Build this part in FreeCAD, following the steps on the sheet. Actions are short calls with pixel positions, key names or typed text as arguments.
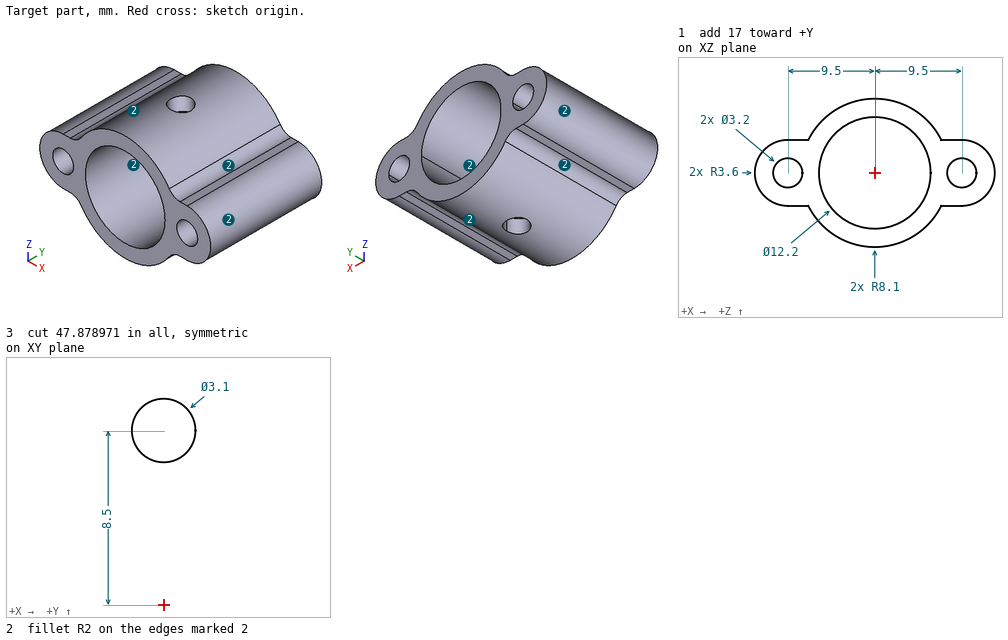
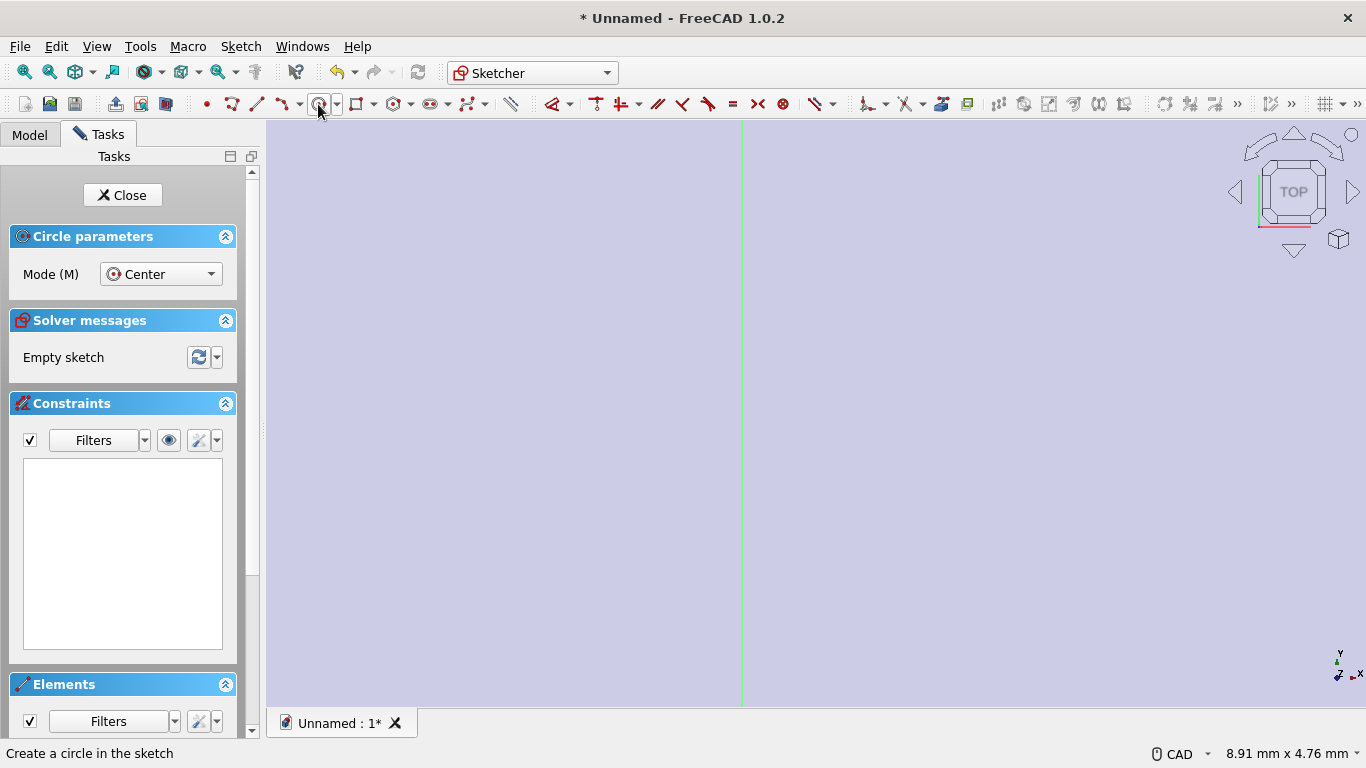
click(742, 407)
click(878, 272)
key(Escape)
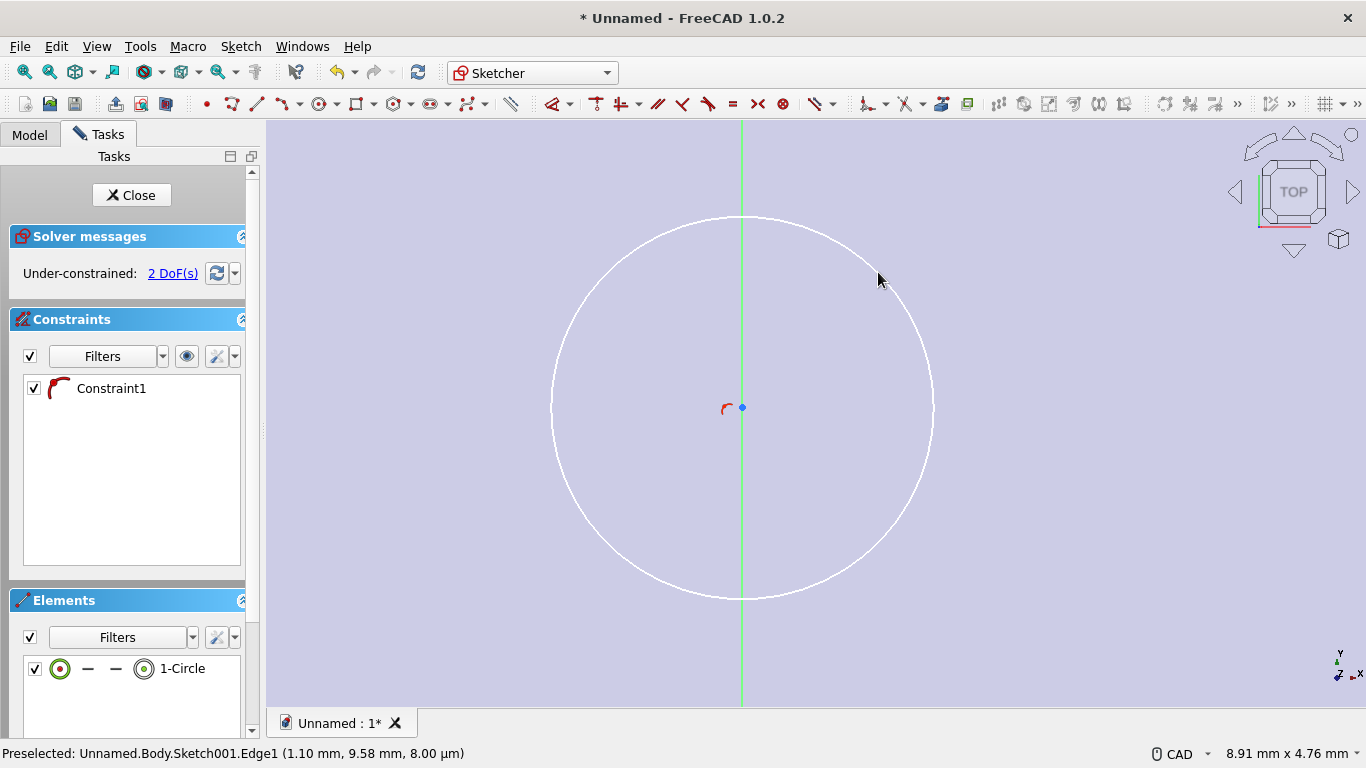
click(877, 272)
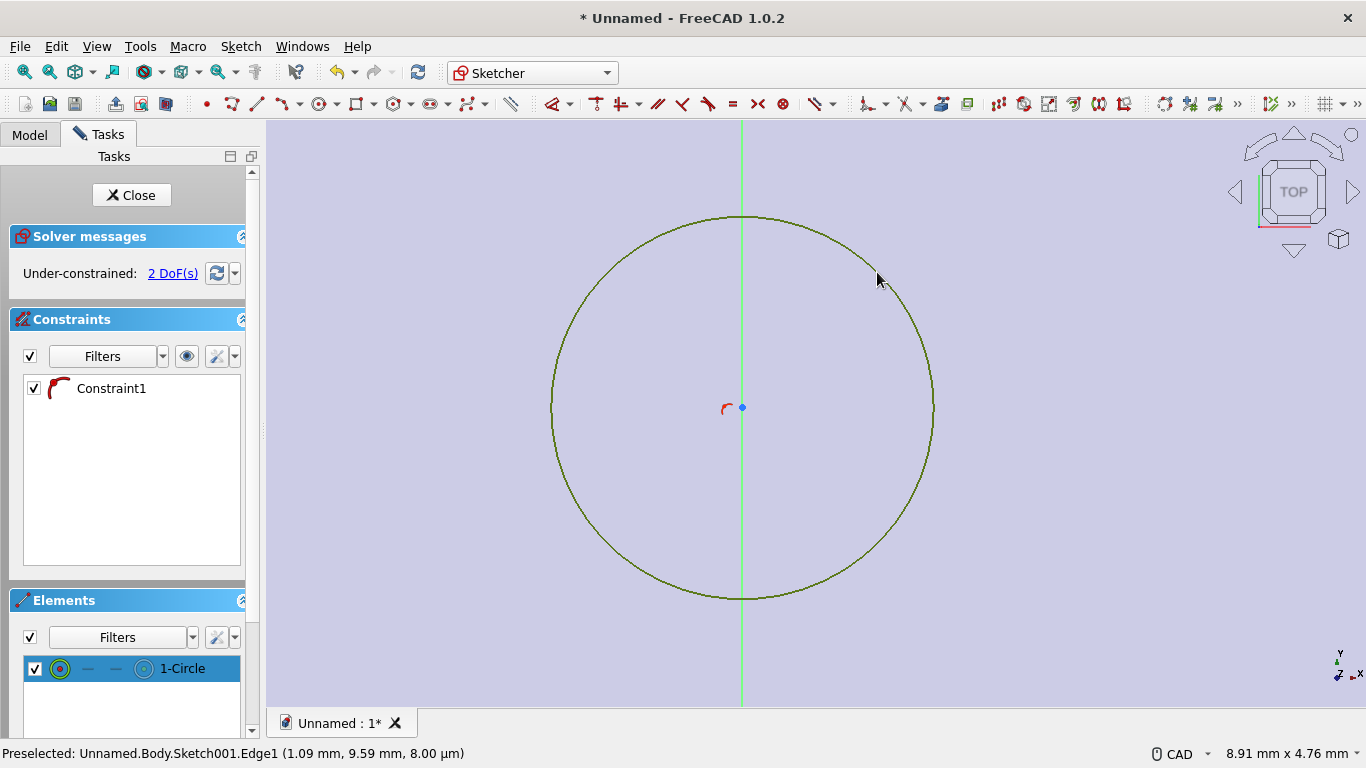
key(k)
key(o)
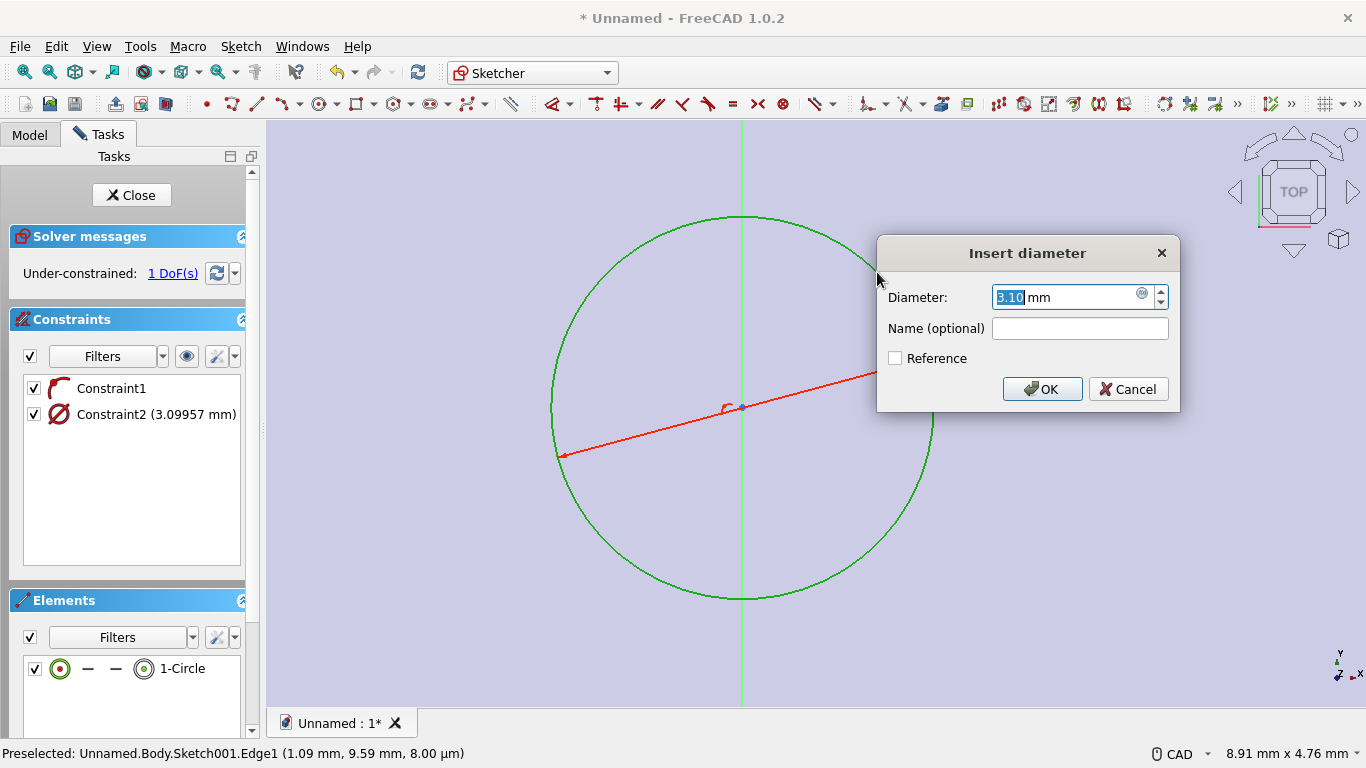
text(3.1)
key(Return)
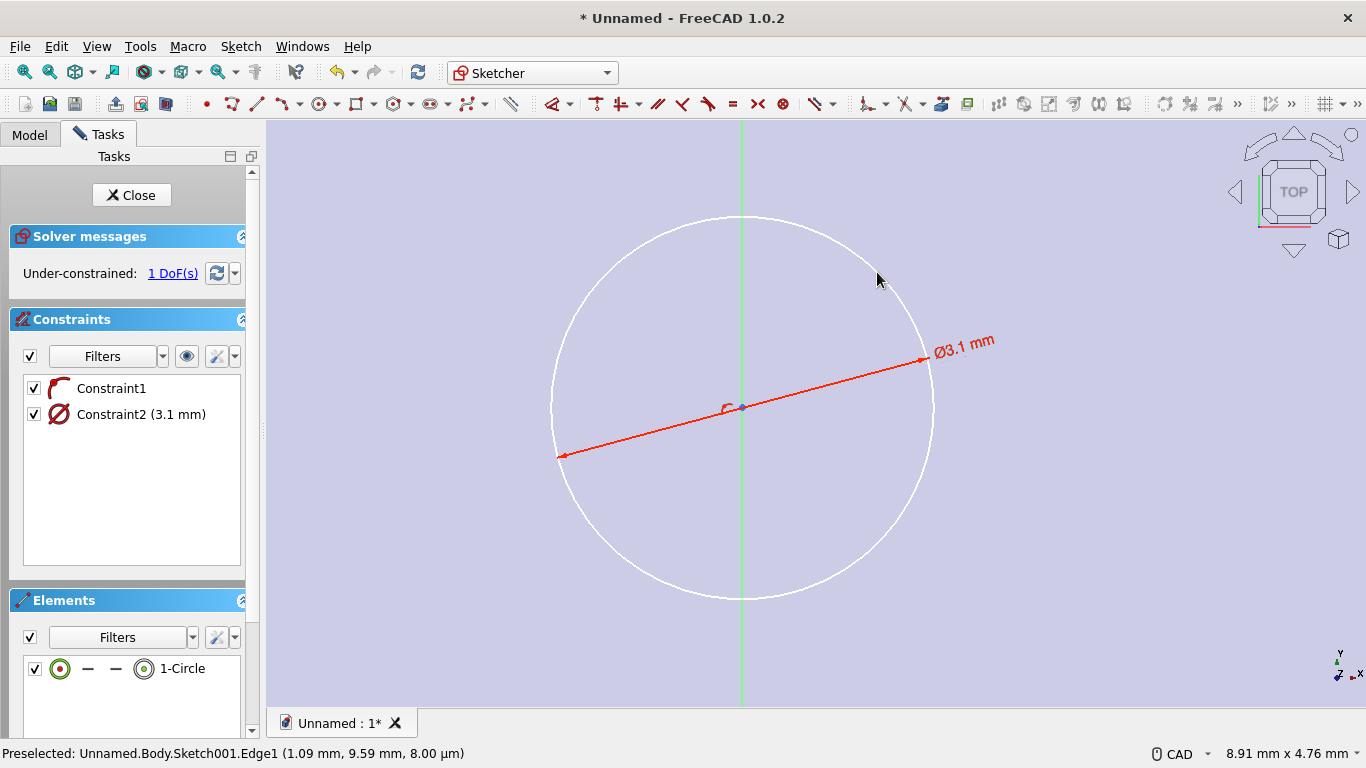
click(742, 408)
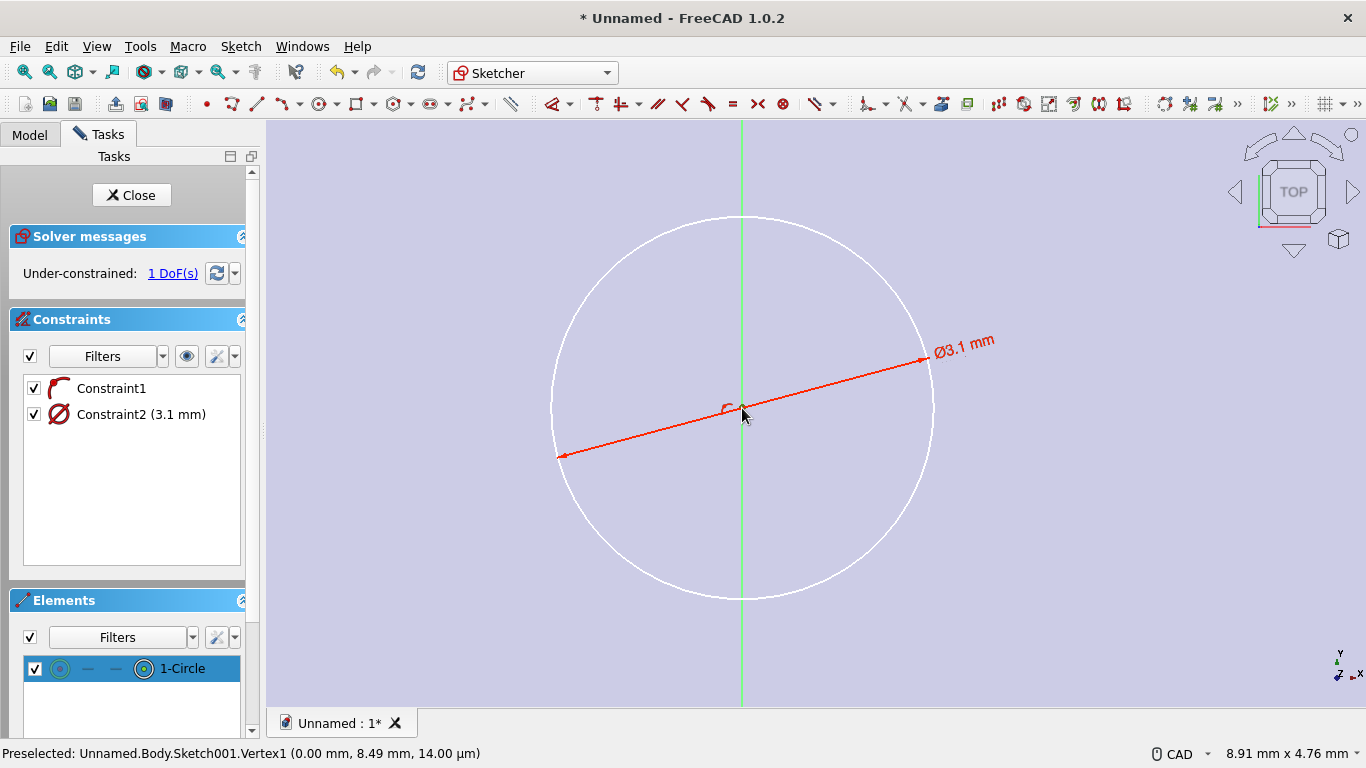
key(i)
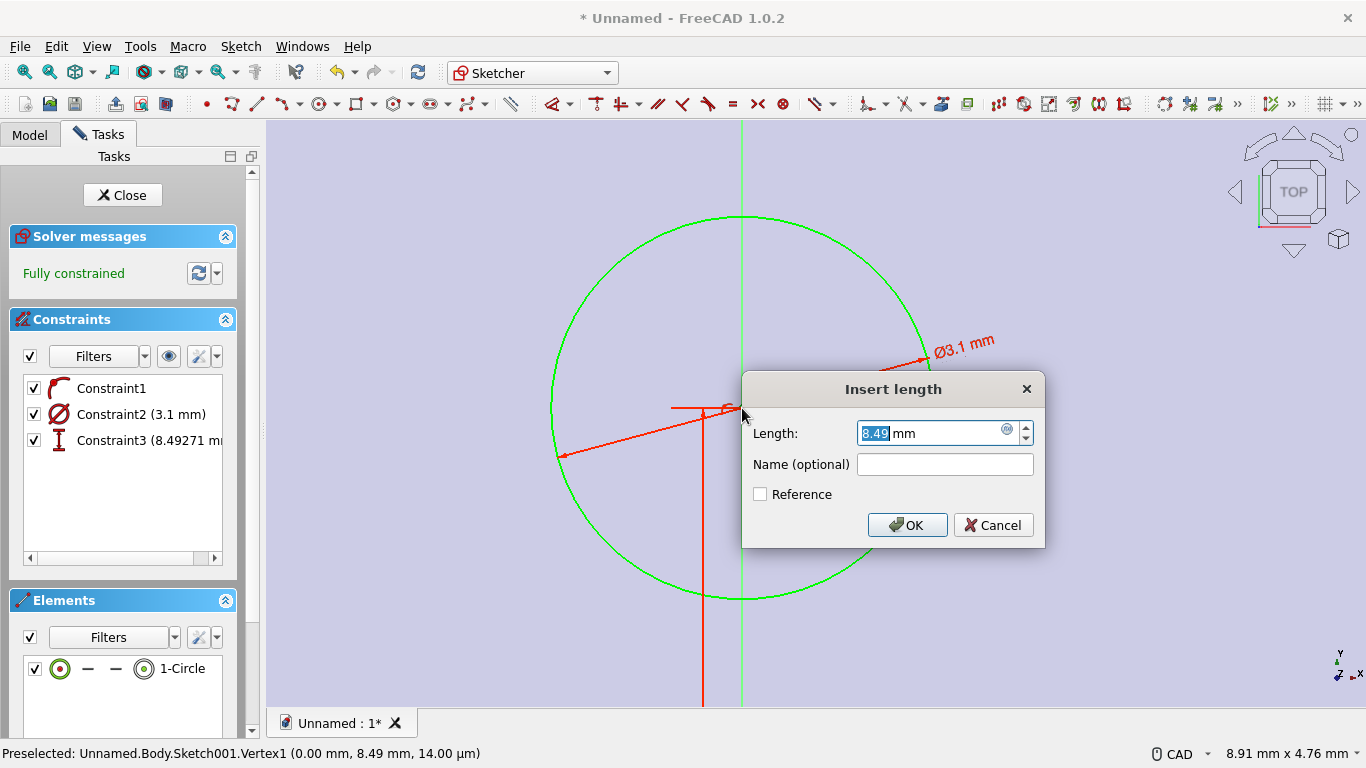
text(8.5)
key(Return)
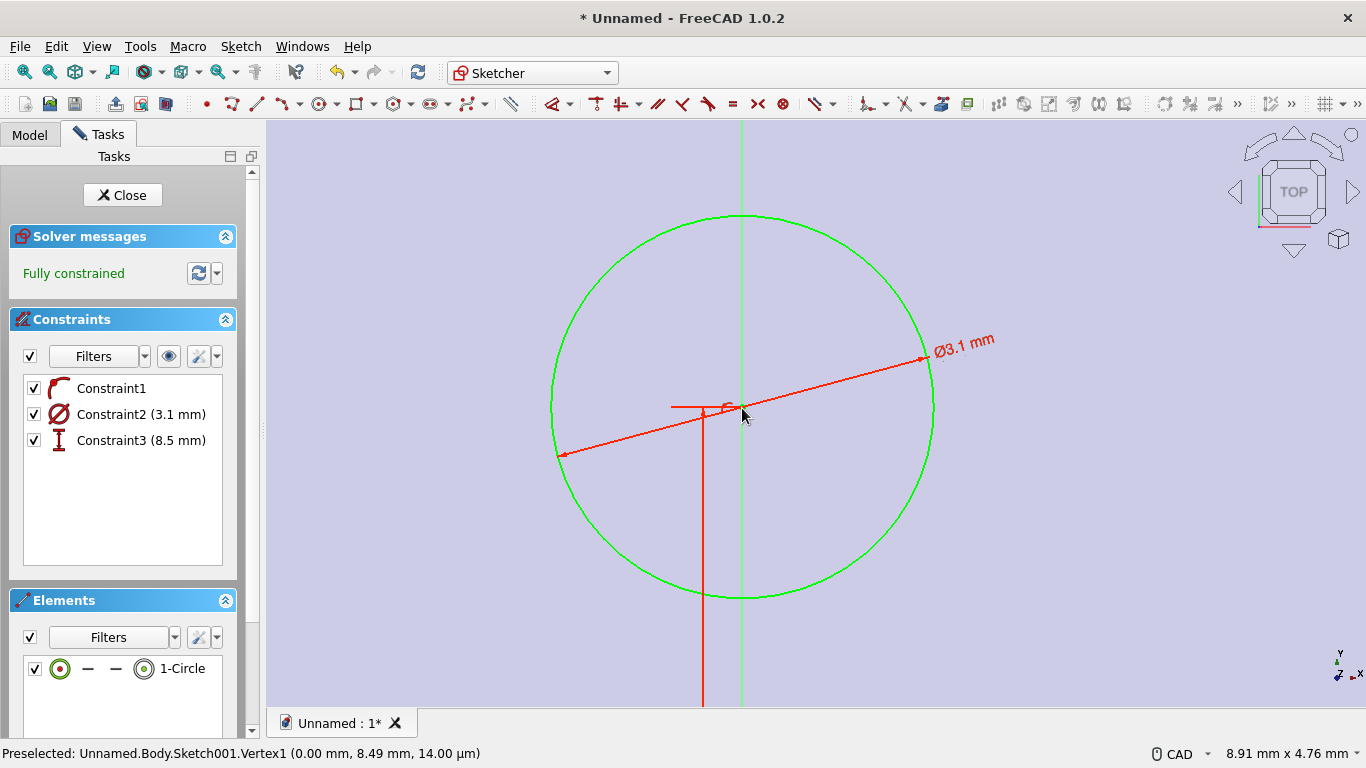
click(123, 195)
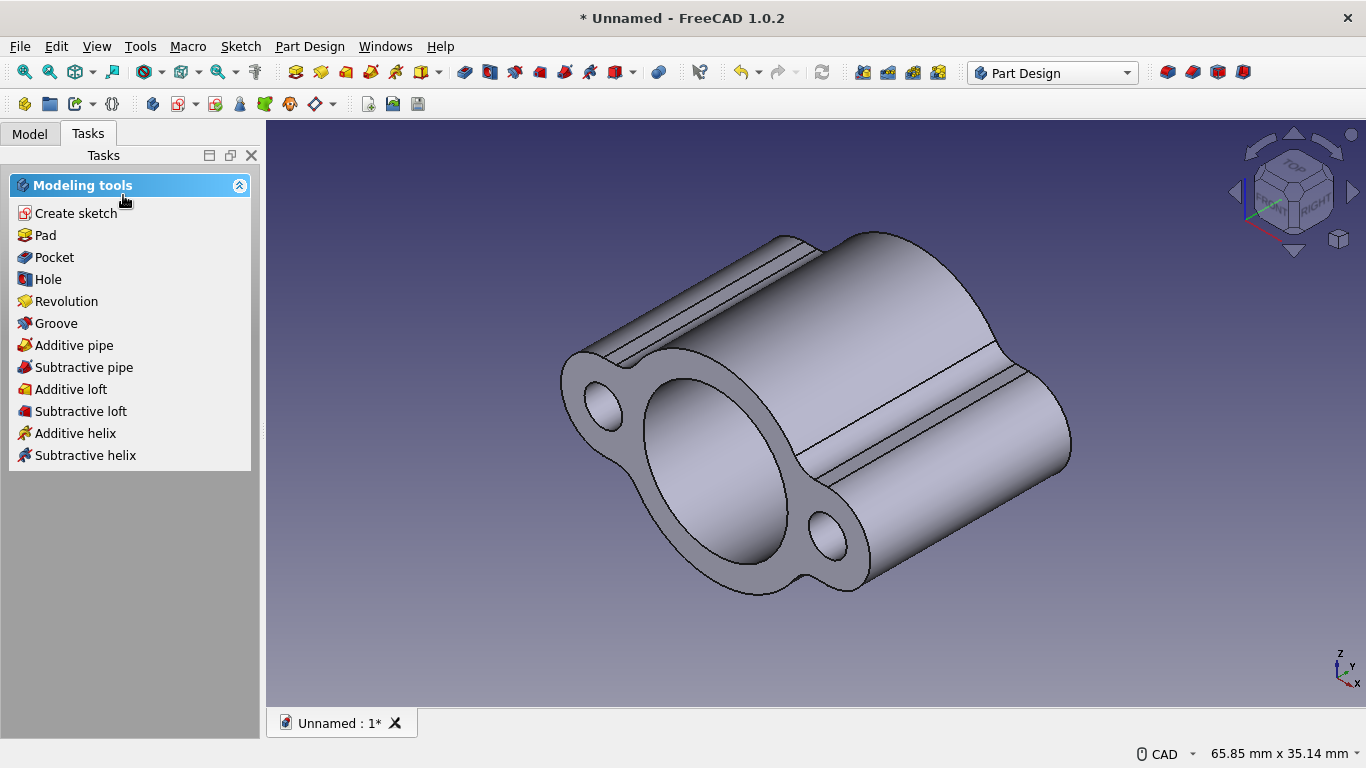
click(465, 72)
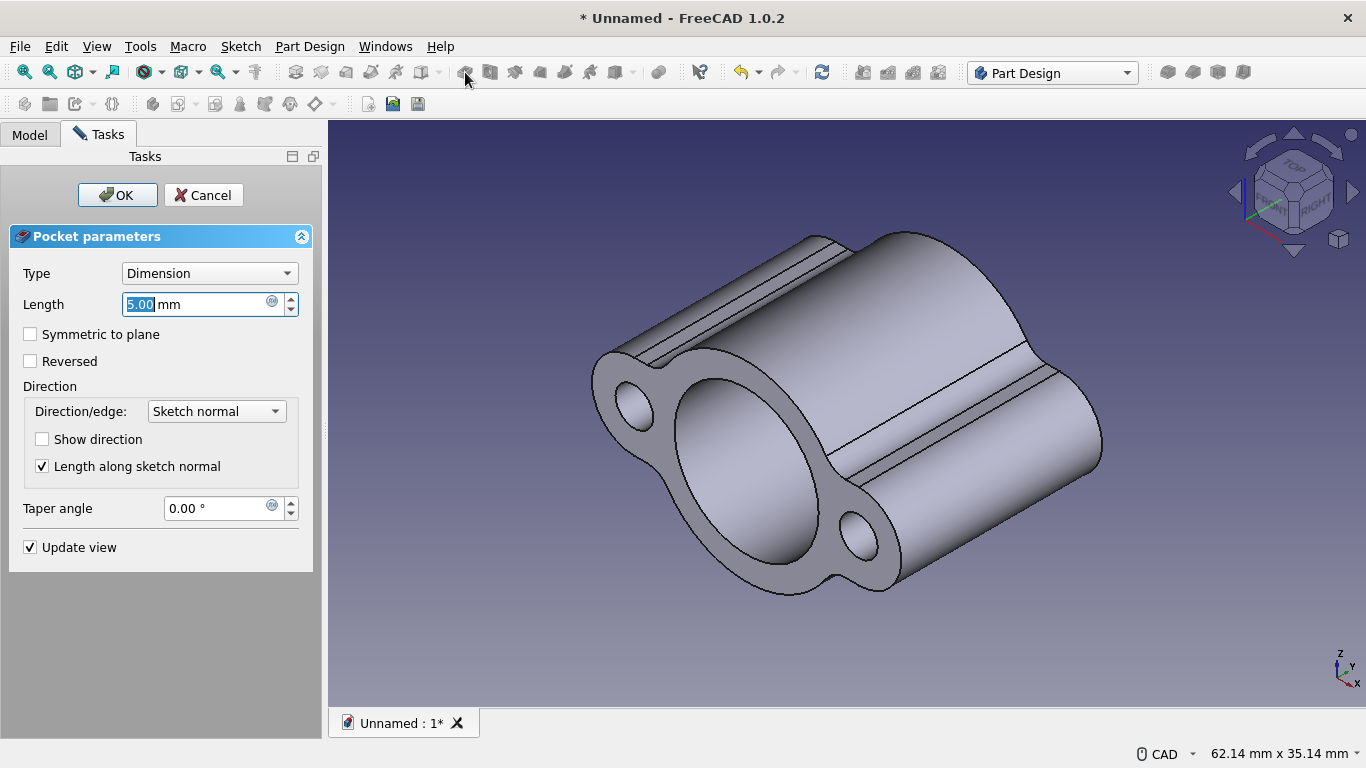
text(47.878971)
key(Tab)